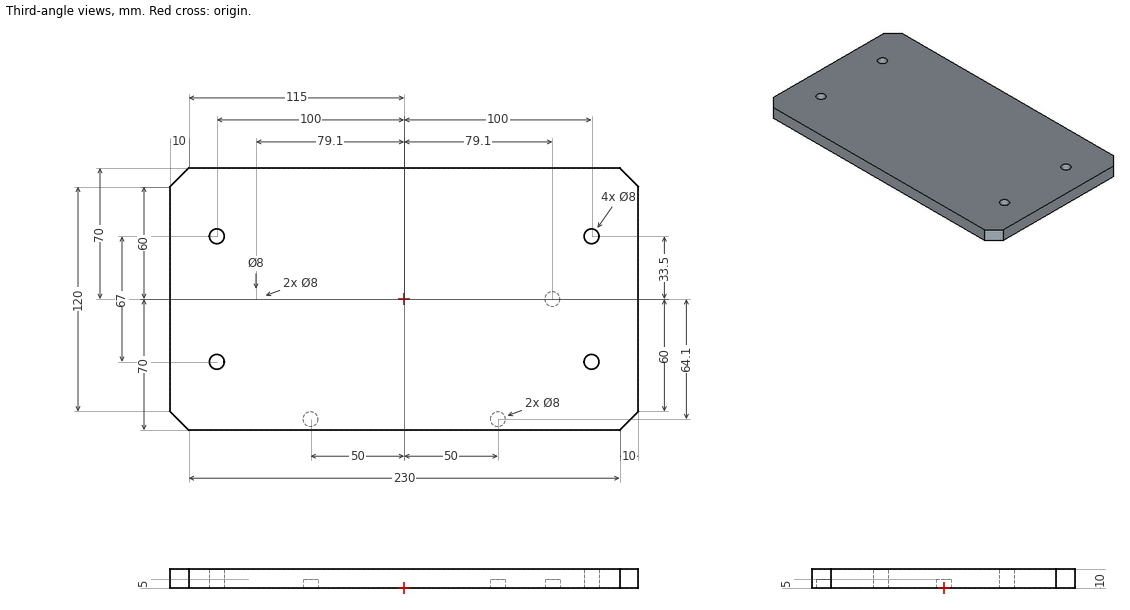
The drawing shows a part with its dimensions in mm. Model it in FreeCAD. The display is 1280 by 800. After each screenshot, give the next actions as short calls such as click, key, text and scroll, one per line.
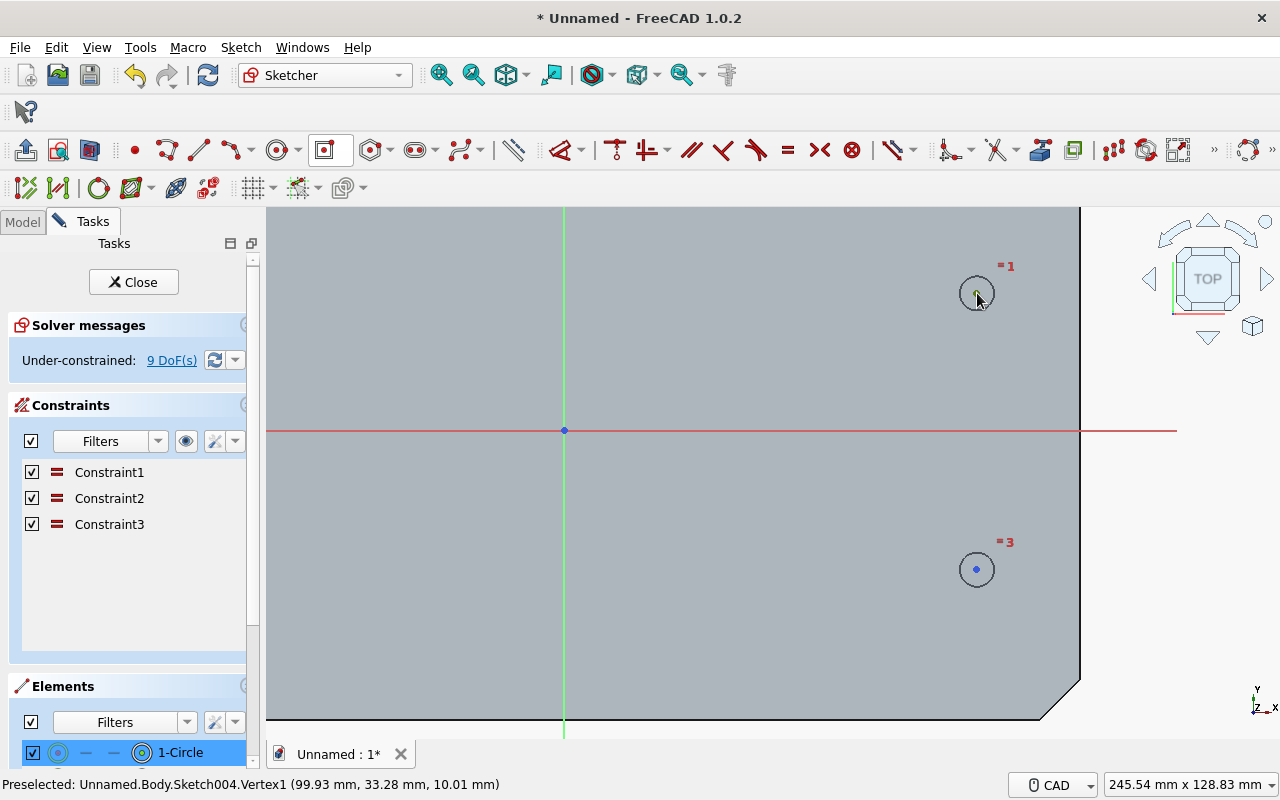
scroll(990, 559, down, 2)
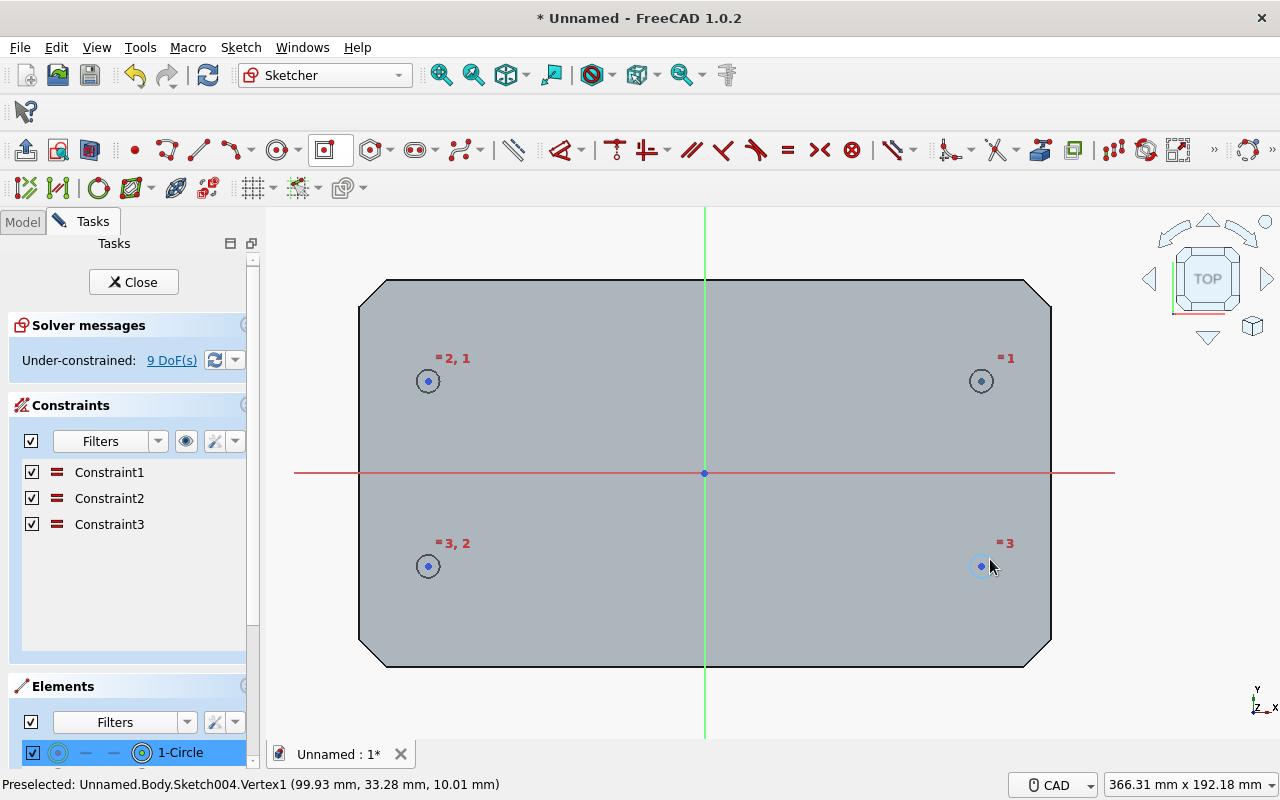
click(428, 381)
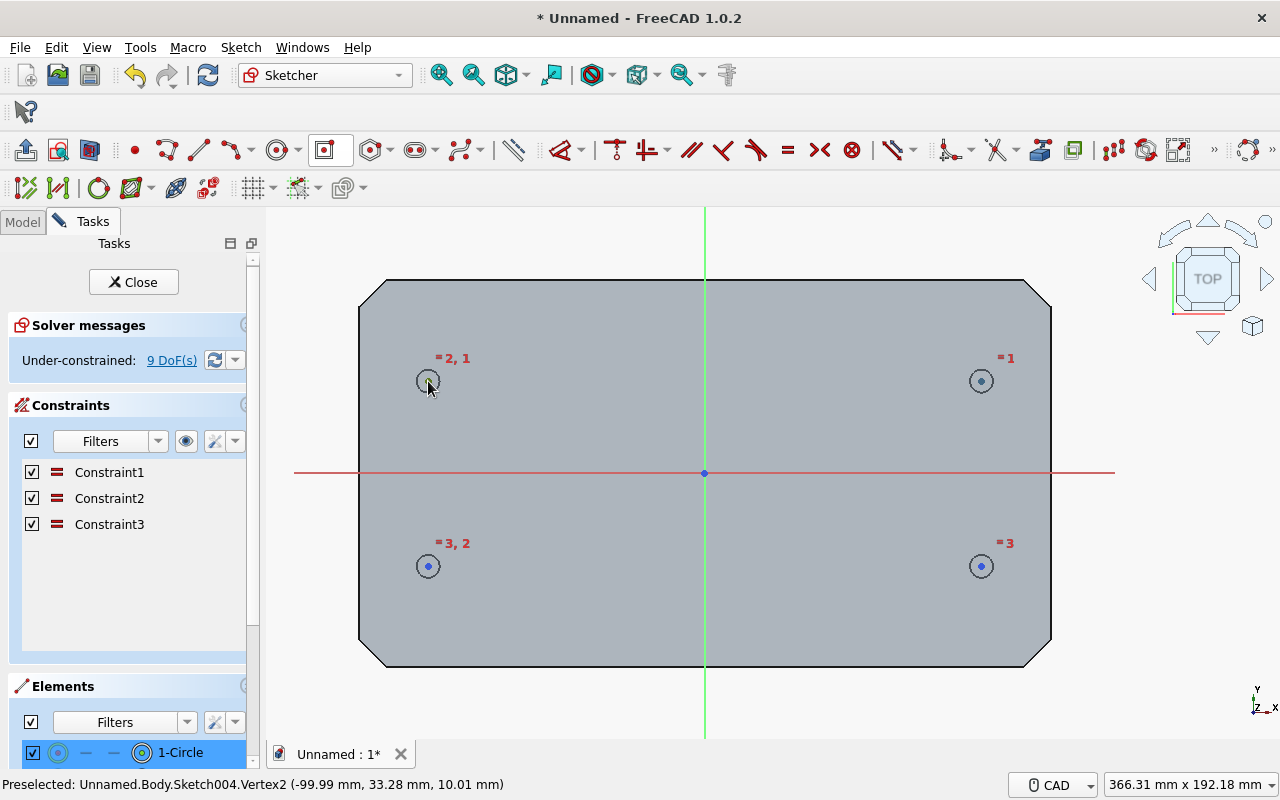
key(h)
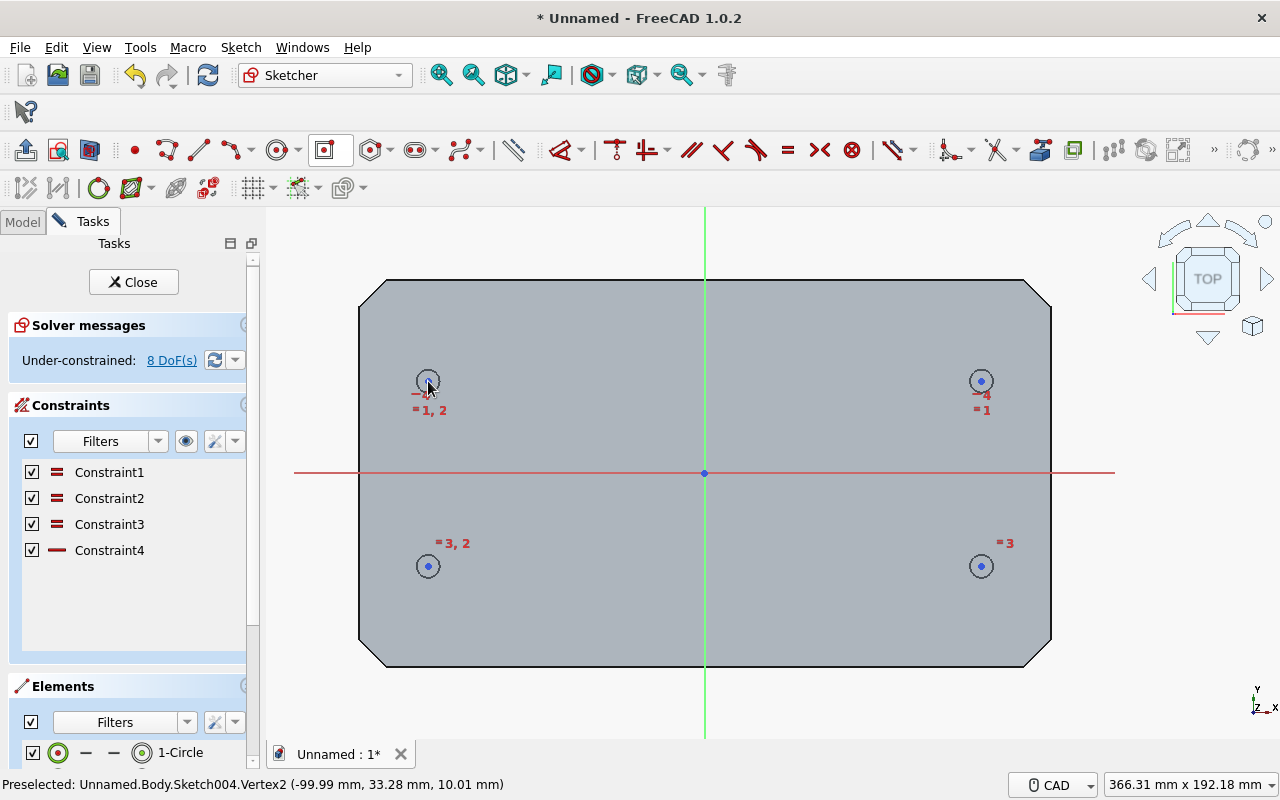
click(428, 381)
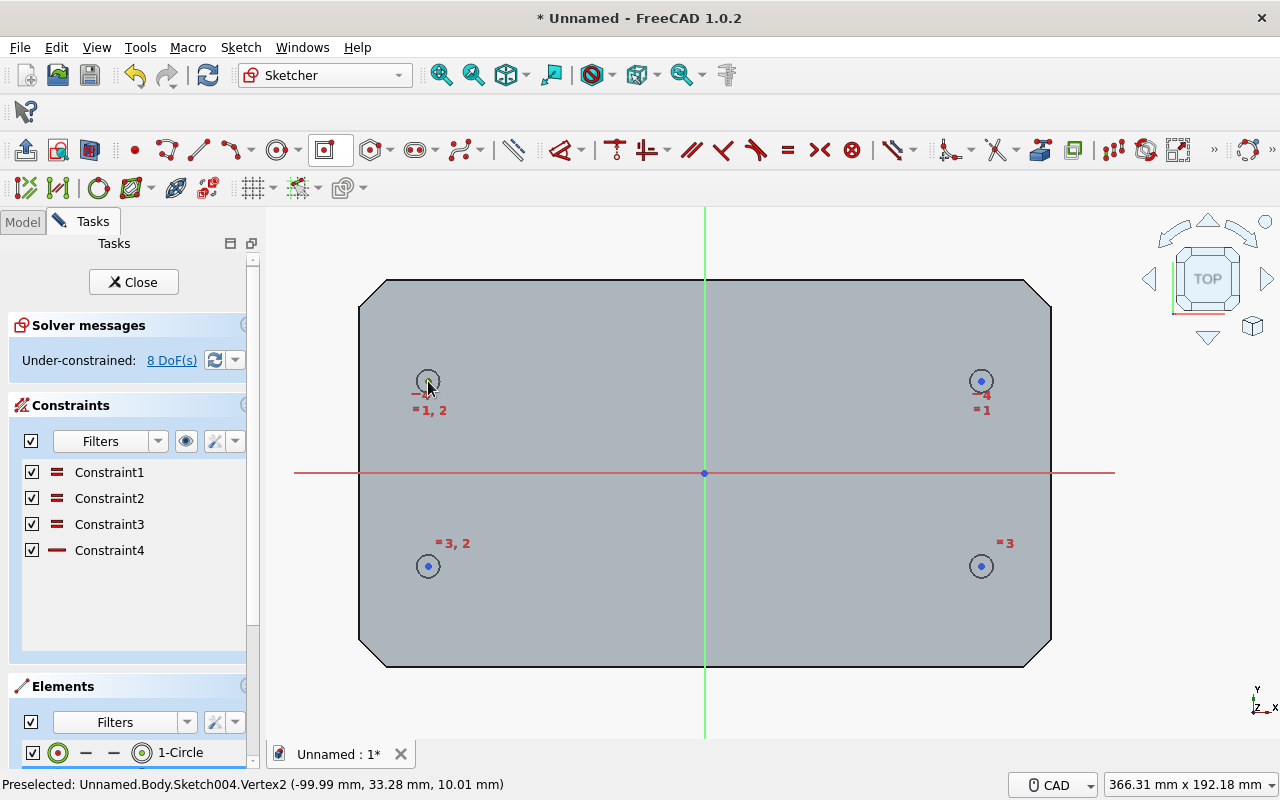
click(428, 566)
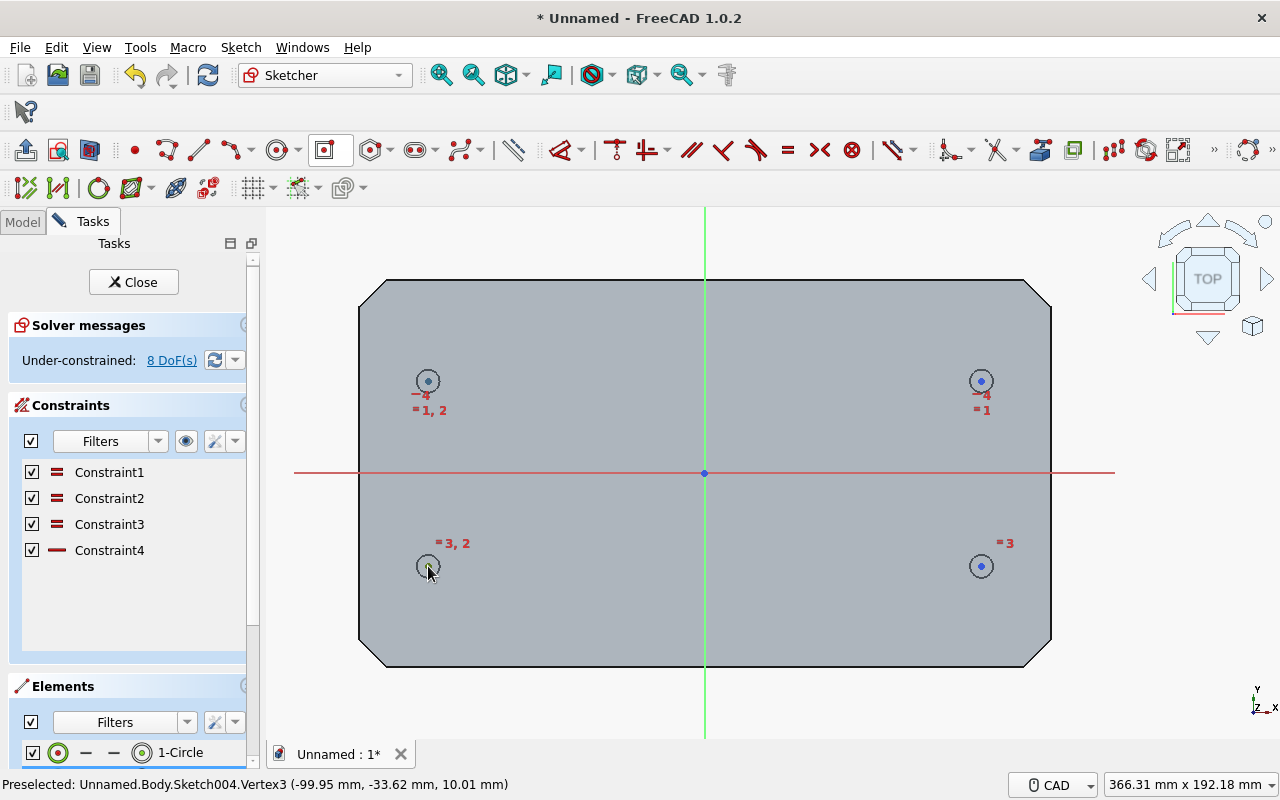
key(v)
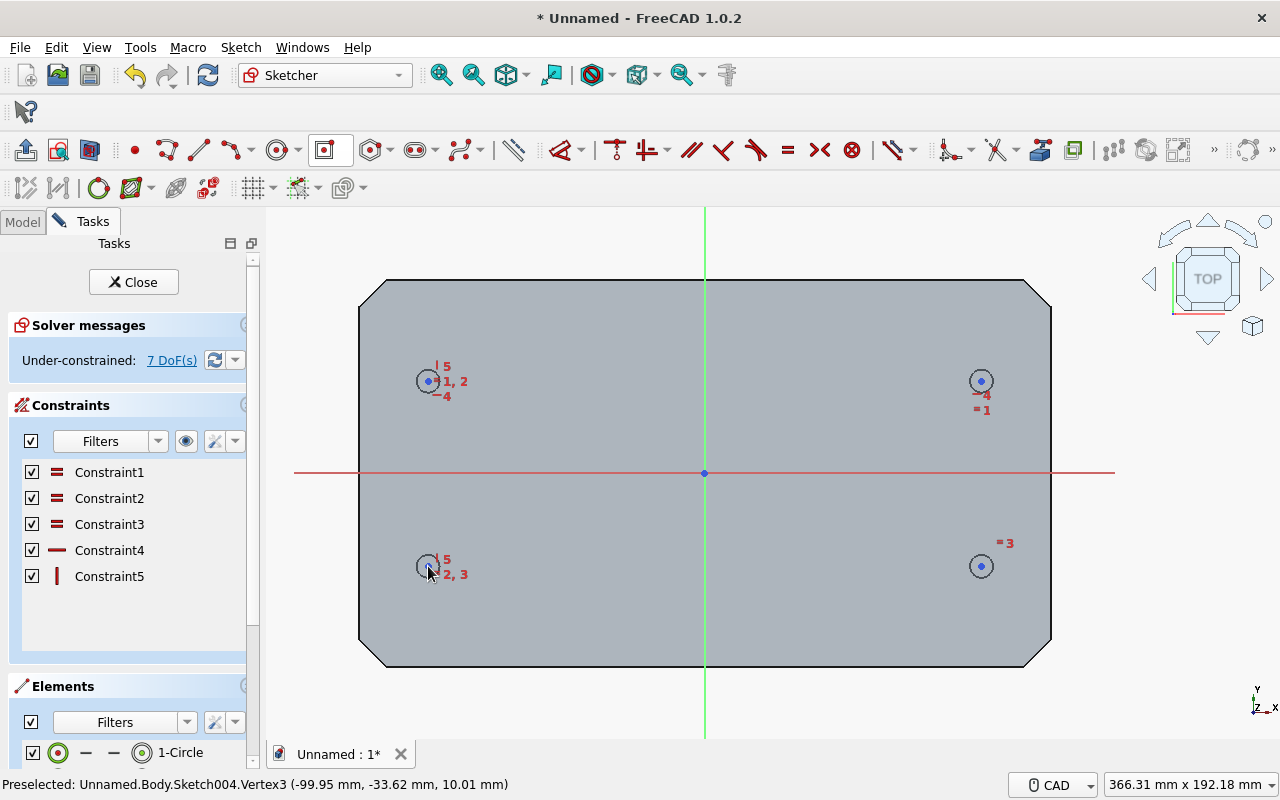
click(981, 381)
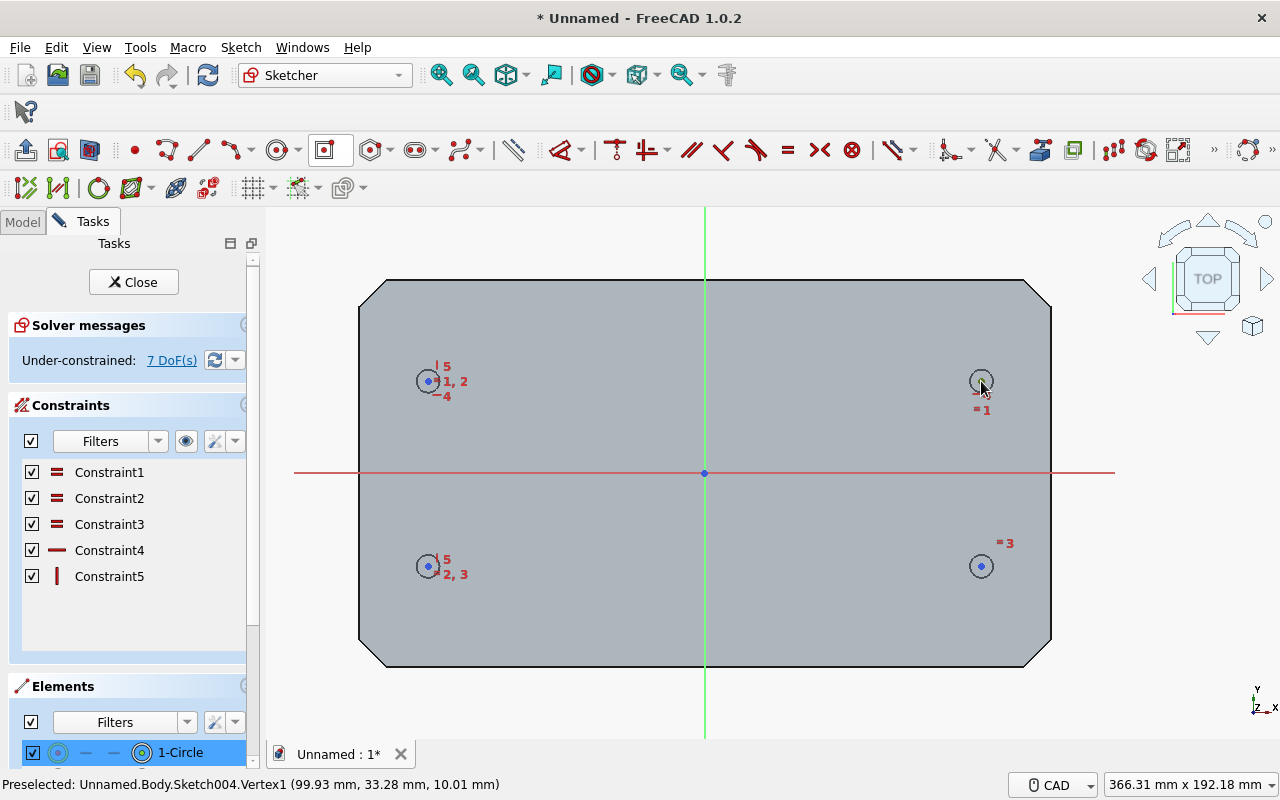
click(981, 566)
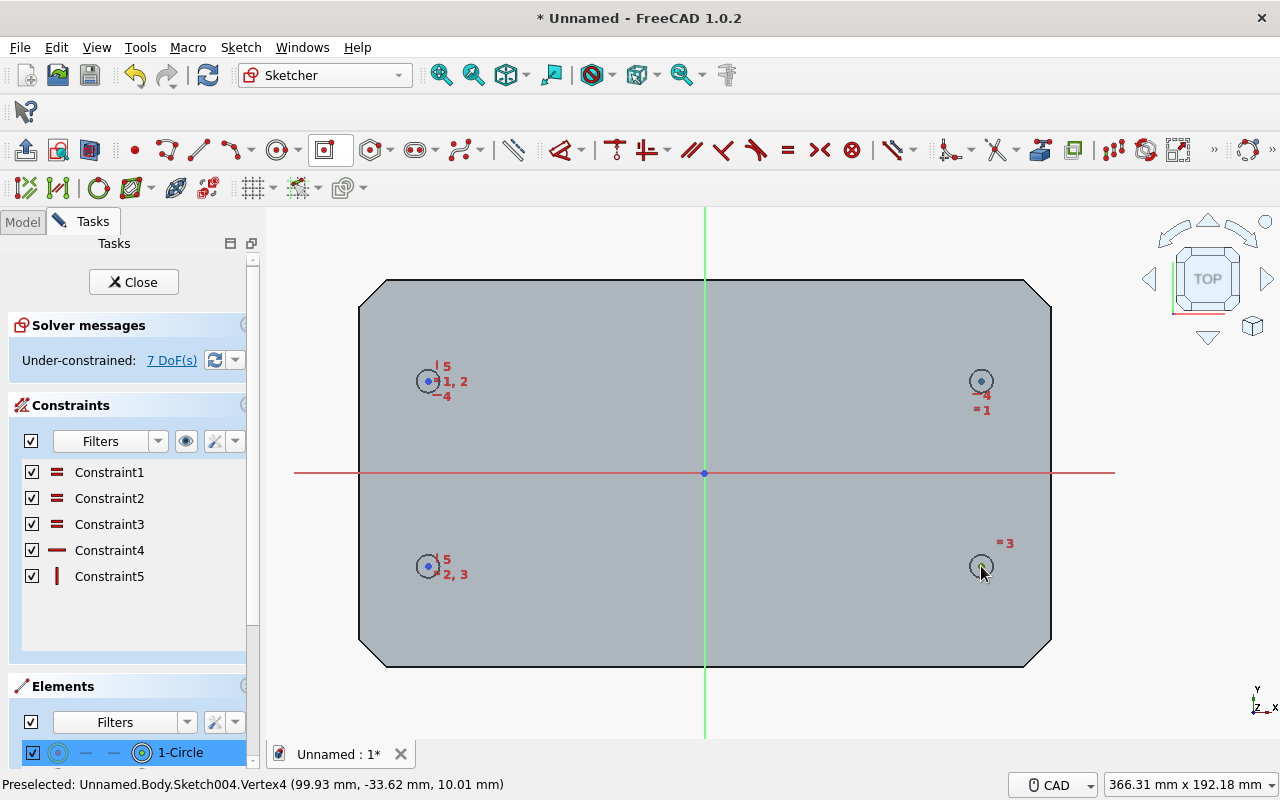
click(670, 150)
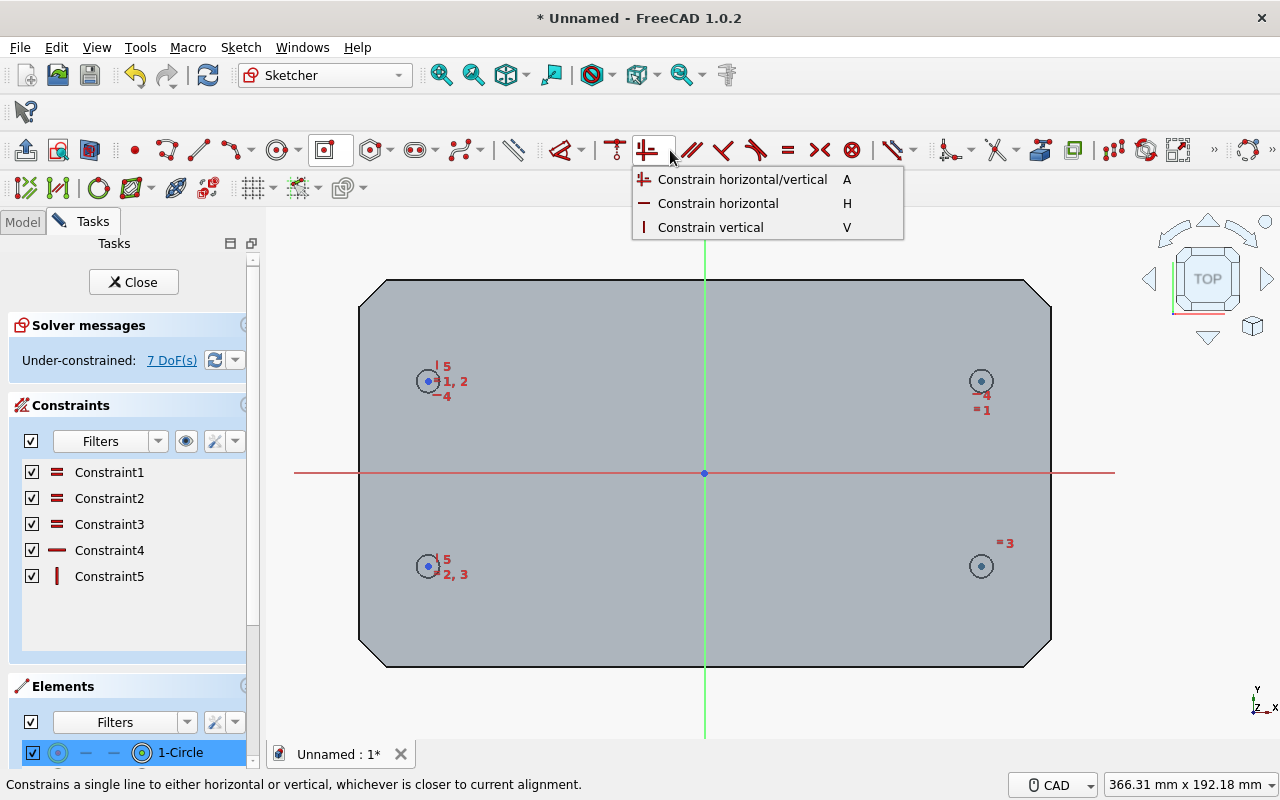
click(768, 227)